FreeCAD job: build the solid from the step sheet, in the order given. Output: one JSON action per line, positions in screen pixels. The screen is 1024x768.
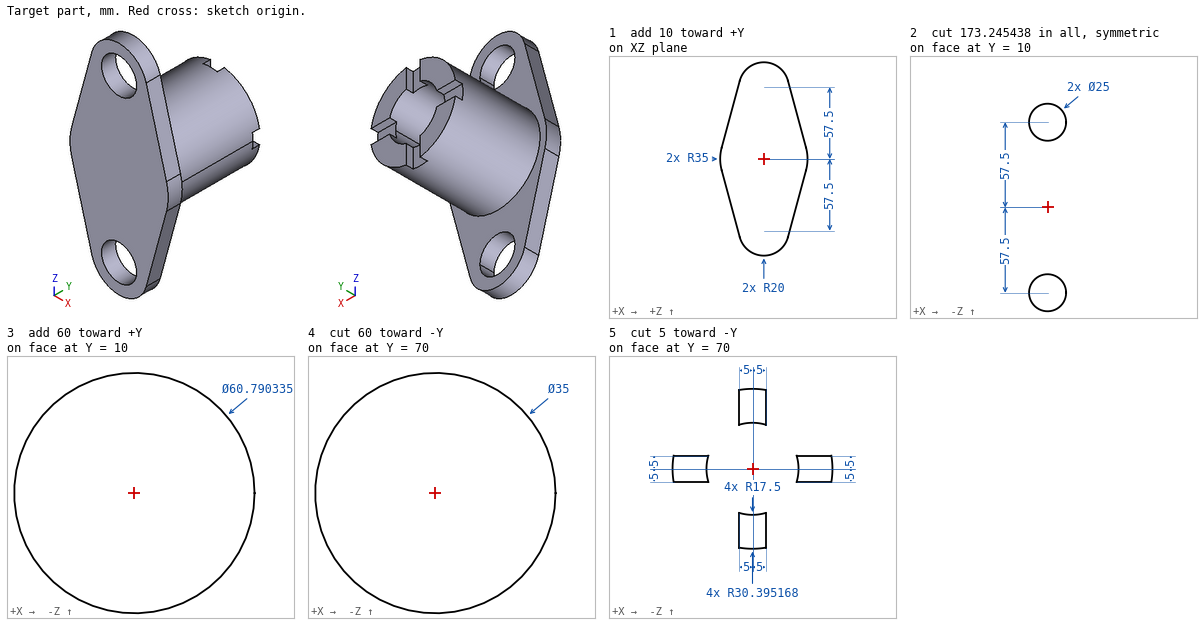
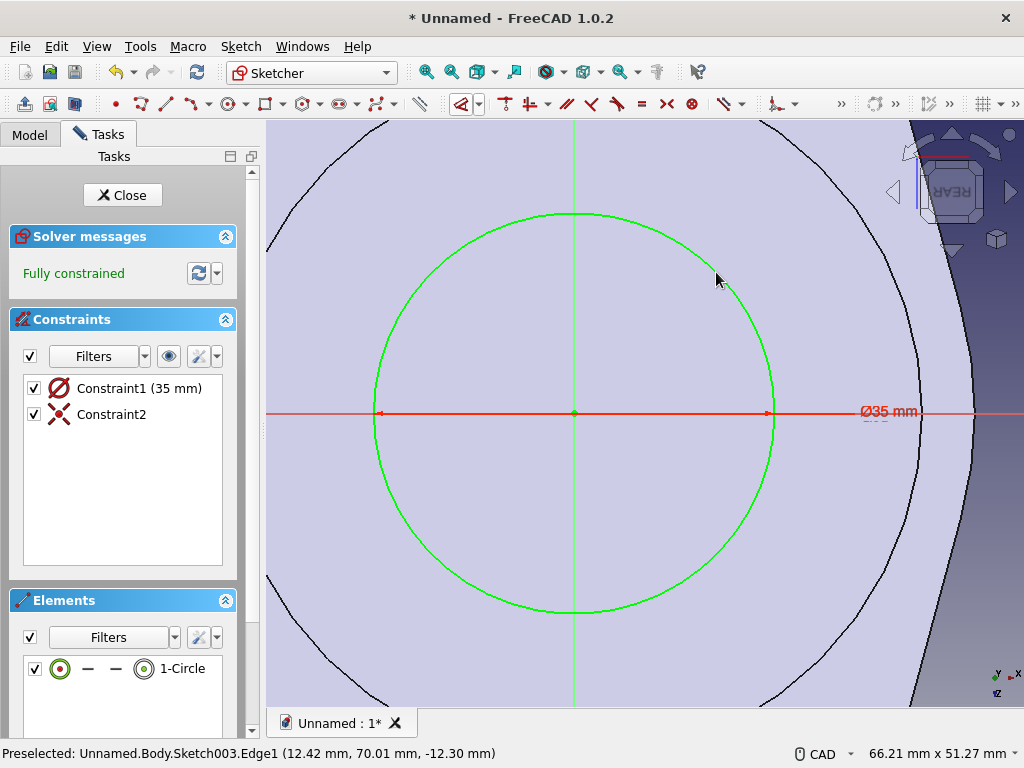
{"action": "left_click", "coordinate": [123, 195]}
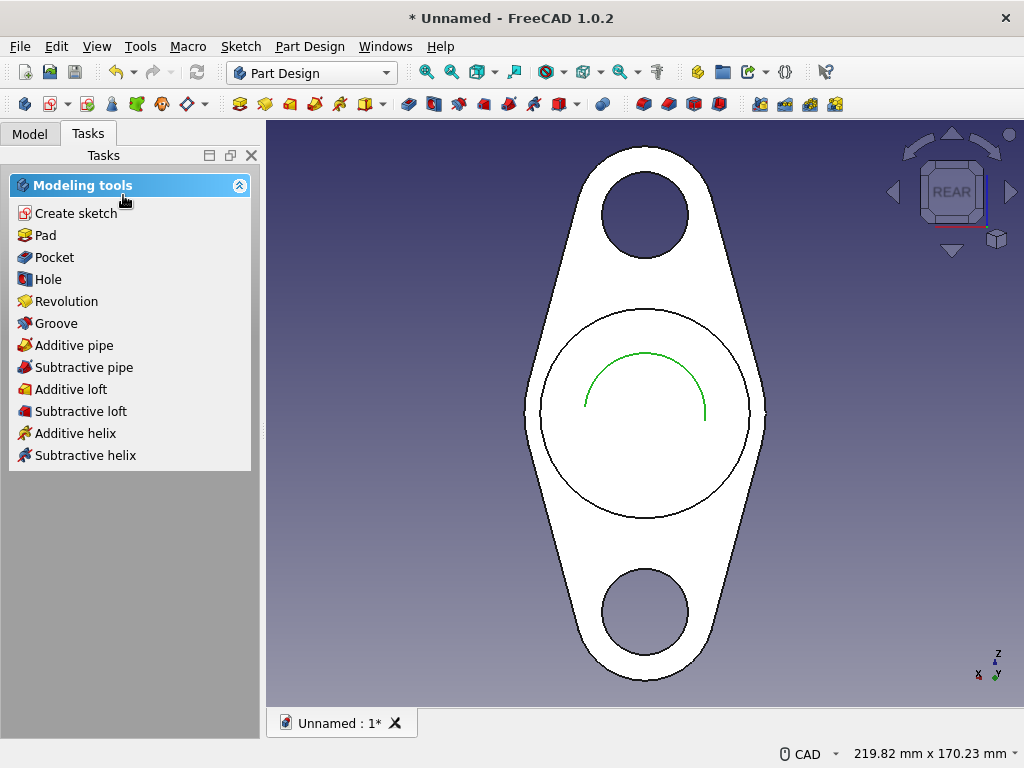
{"action": "left_click", "coordinate": [409, 104]}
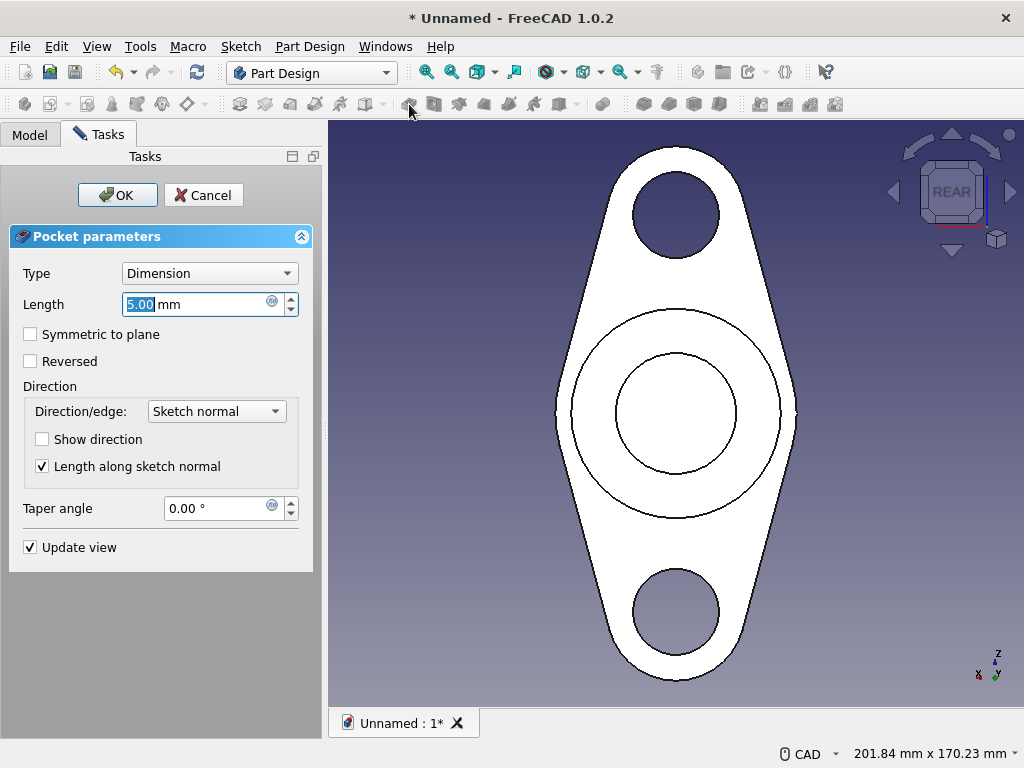
{"action": "type", "text": "60"}
{"action": "key", "text": "Tab"}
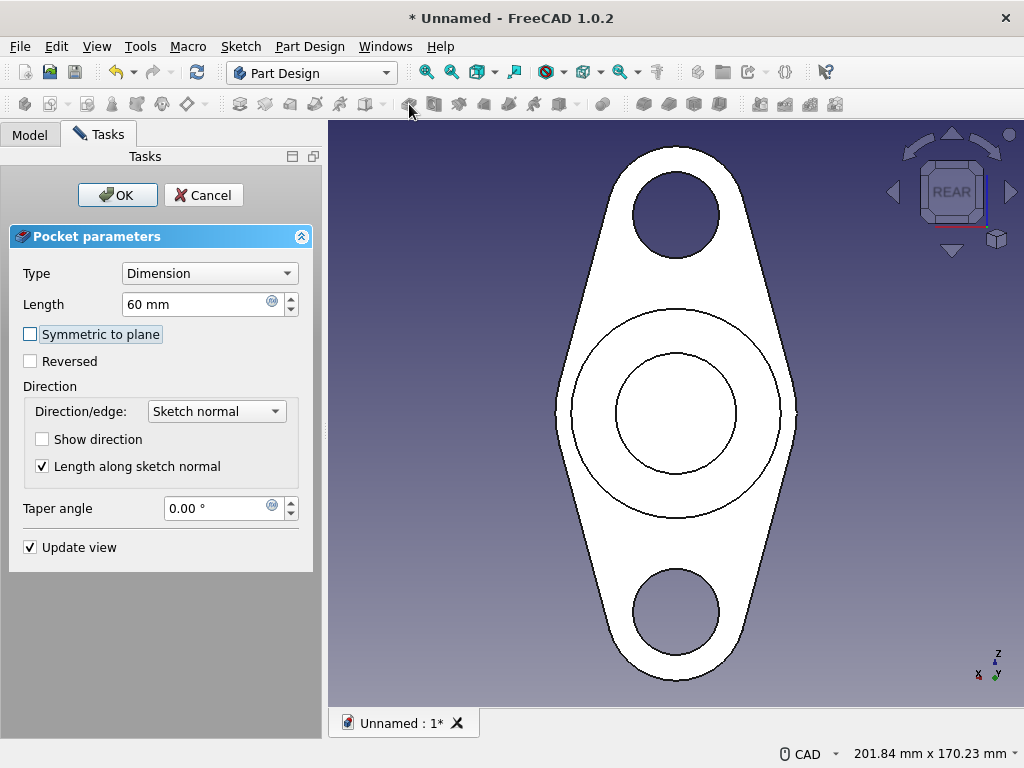
{"action": "left_click", "coordinate": [118, 195]}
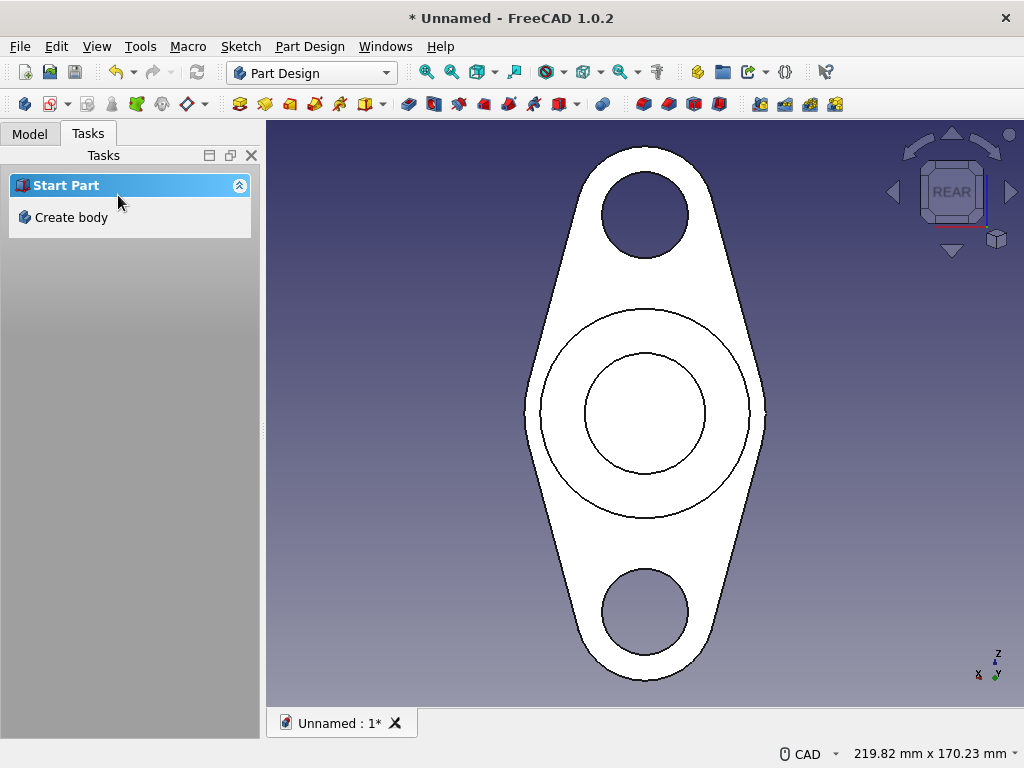
{"action": "left_click", "coordinate": [705, 353]}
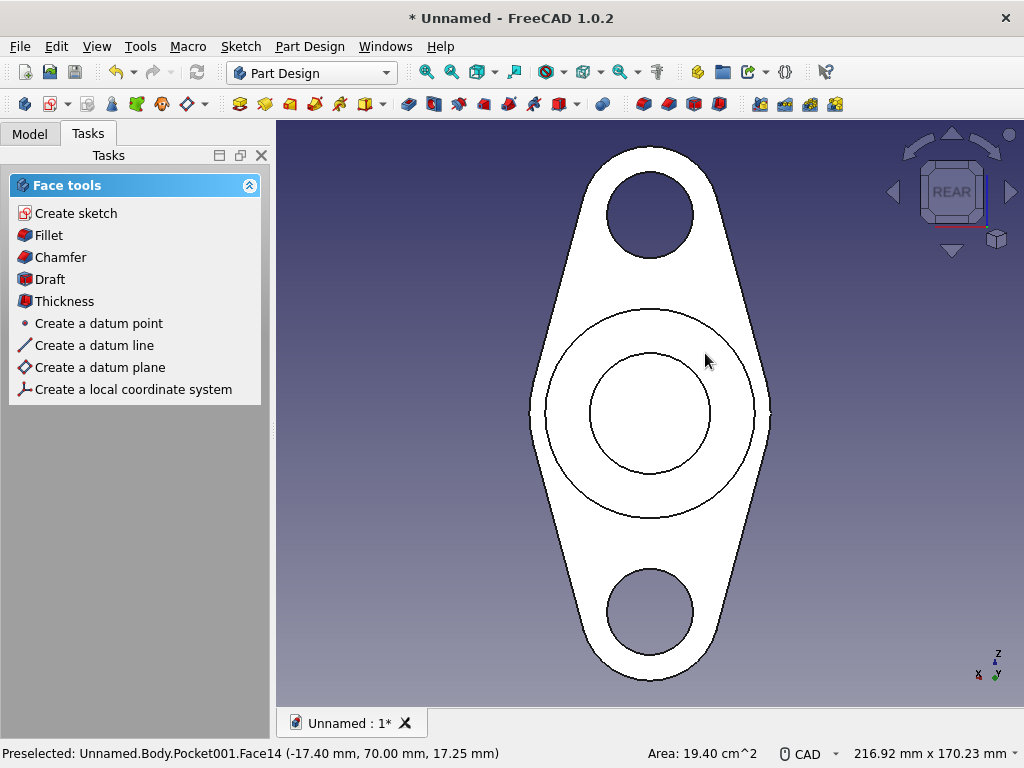
{"action": "left_click", "coordinate": [50, 104]}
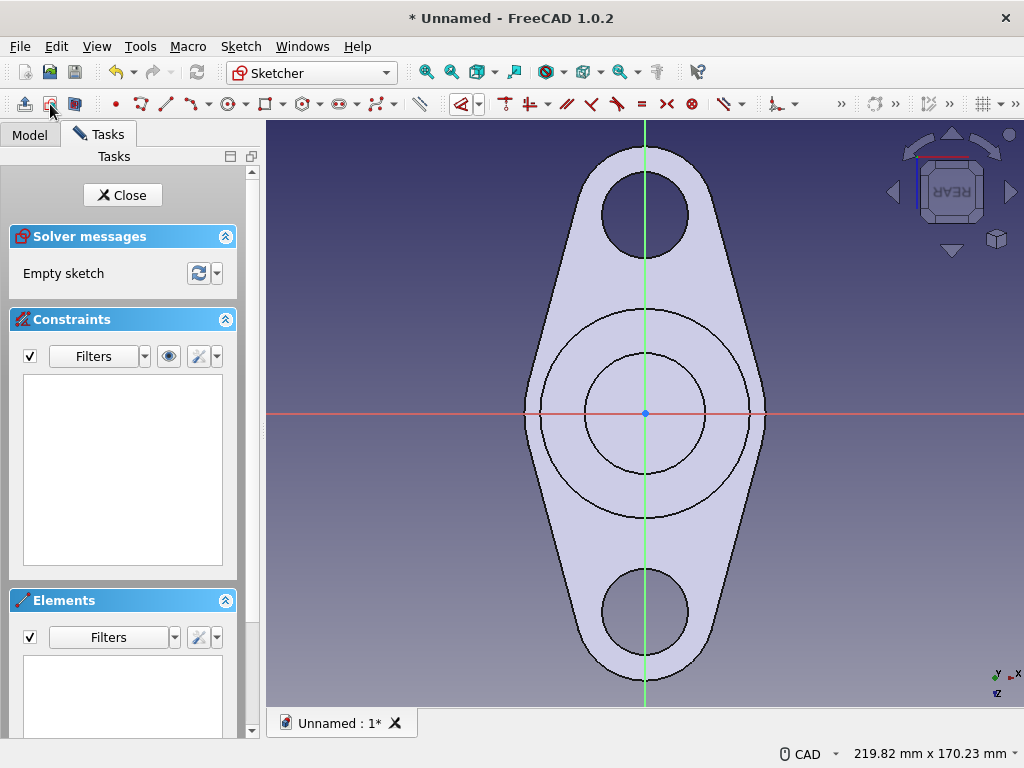
{"action": "scroll", "coordinate": [728, 413], "scroll_direction": "up", "scroll_amount": 3}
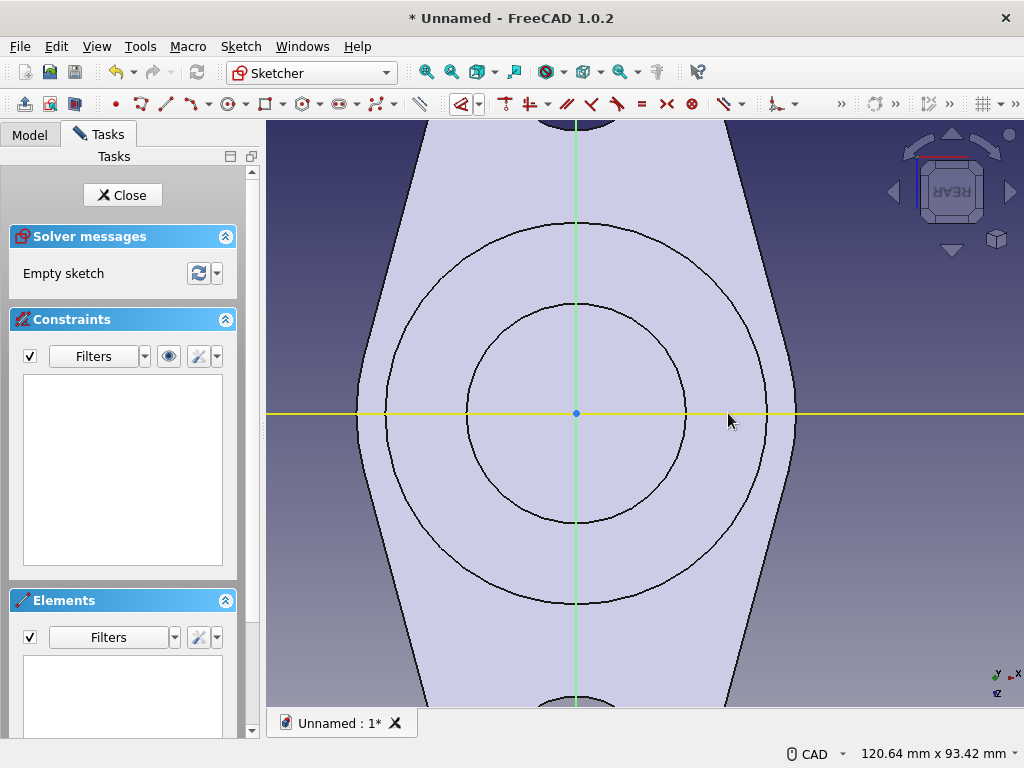
{"action": "left_click", "coordinate": [166, 104]}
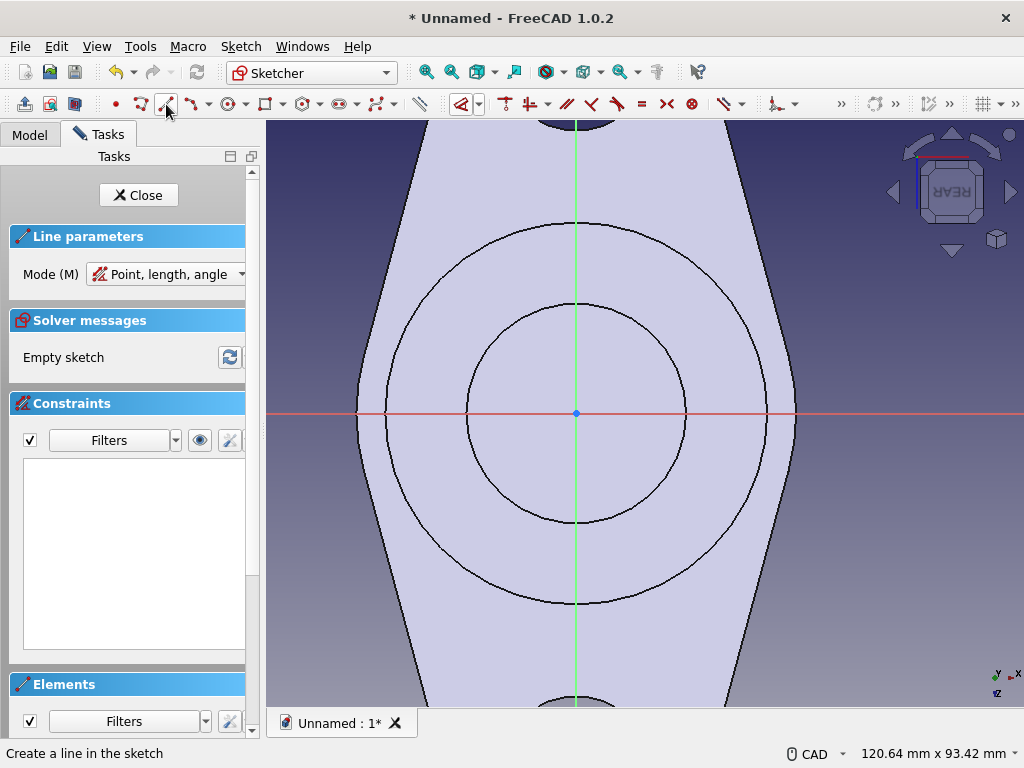
{"action": "left_click", "coordinate": [388, 445]}
{"action": "left_click", "coordinate": [471, 445]}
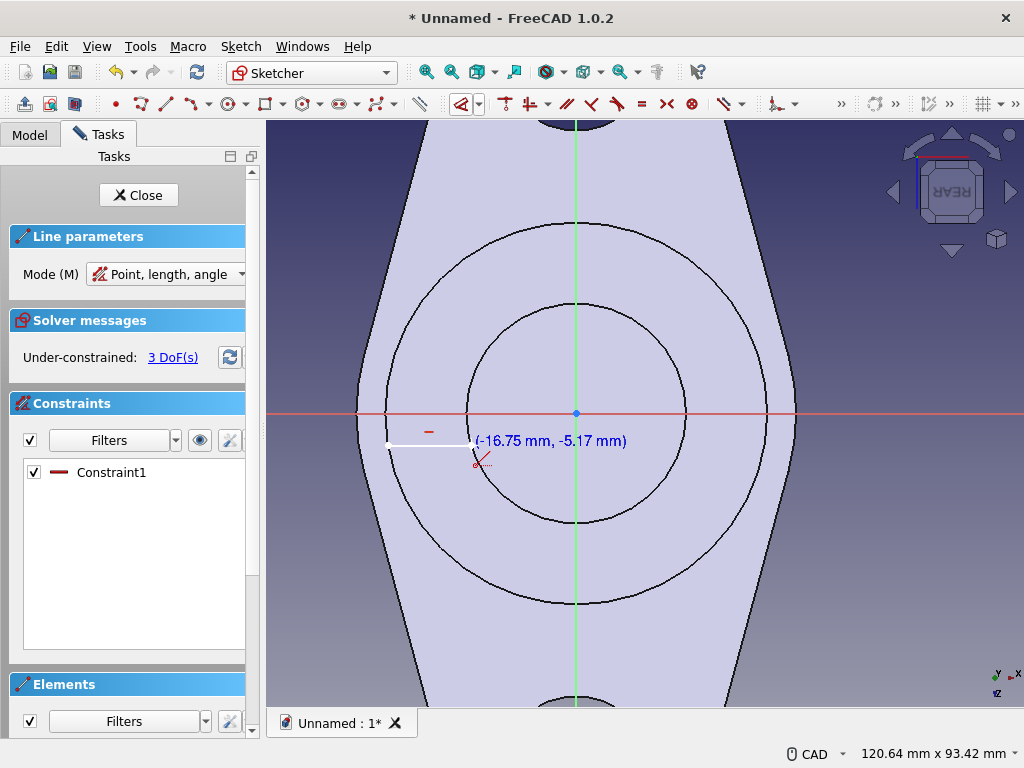
{"action": "left_click", "coordinate": [471, 382]}
{"action": "left_click", "coordinate": [388, 382]}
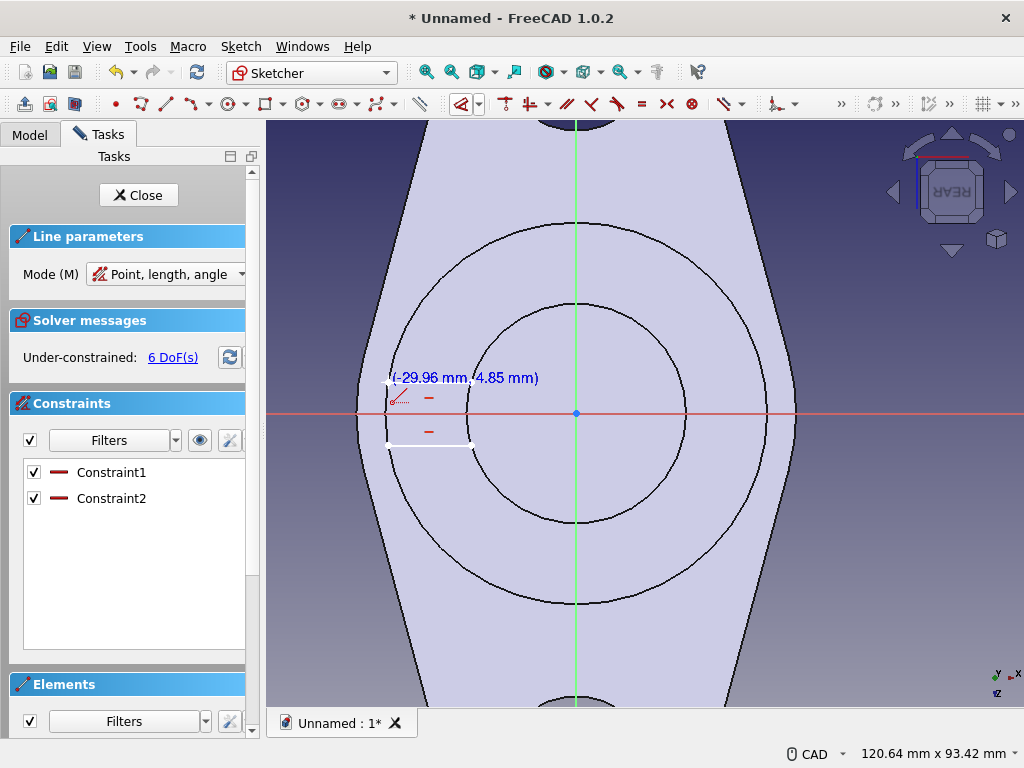
{"action": "left_click", "coordinate": [190, 104]}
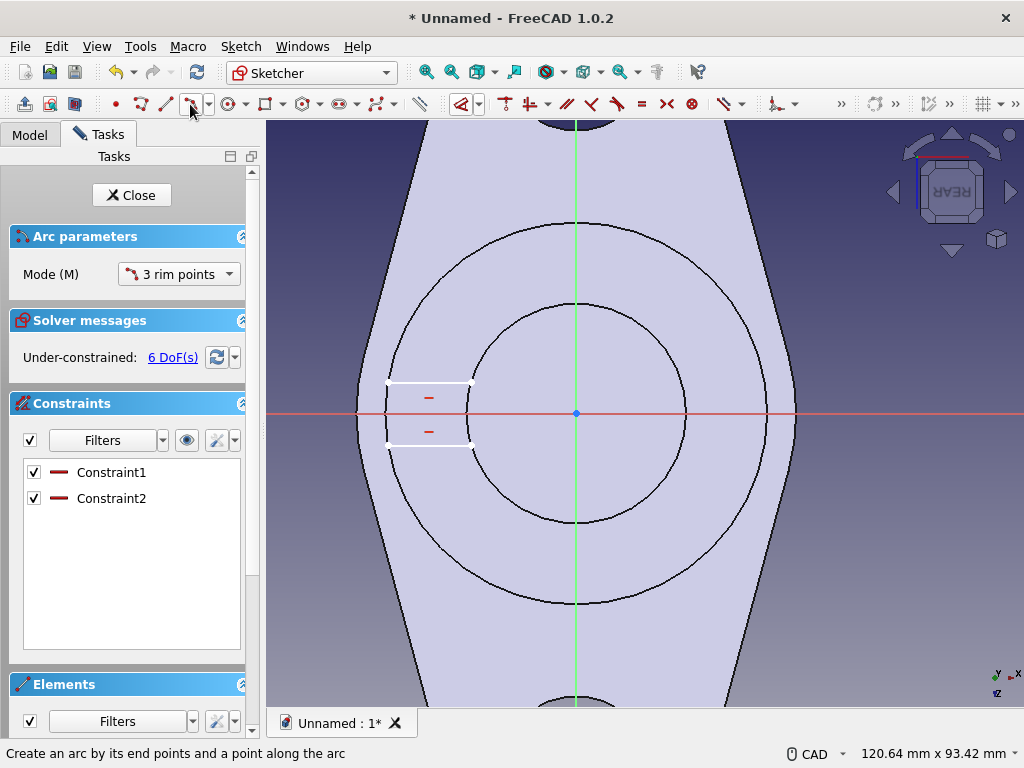
{"action": "left_click", "coordinate": [471, 446]}
{"action": "left_click", "coordinate": [471, 383]}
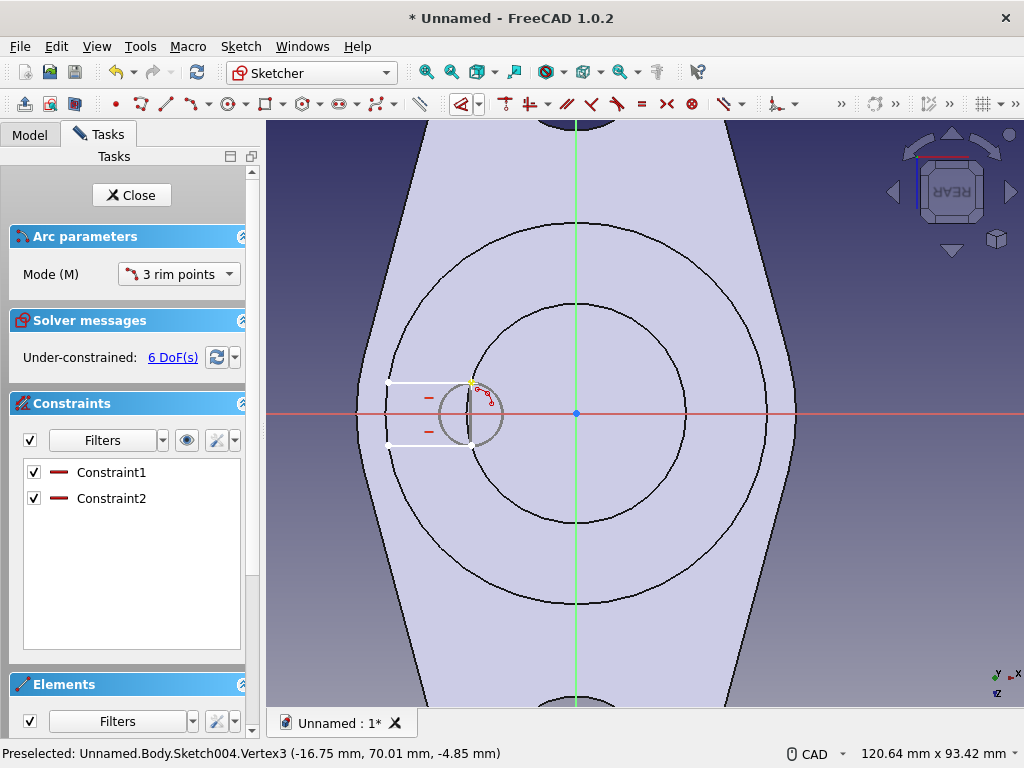
{"action": "scroll", "coordinate": [466, 407], "scroll_direction": "up", "scroll_amount": 7}